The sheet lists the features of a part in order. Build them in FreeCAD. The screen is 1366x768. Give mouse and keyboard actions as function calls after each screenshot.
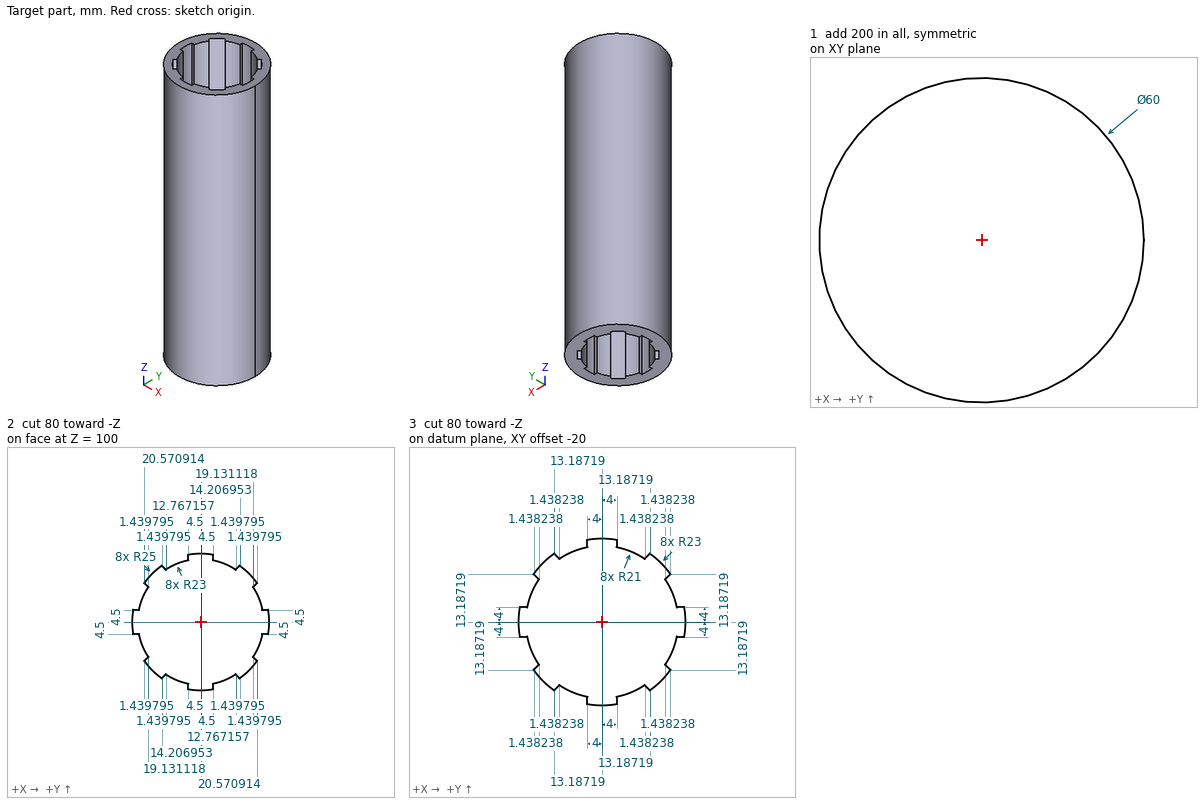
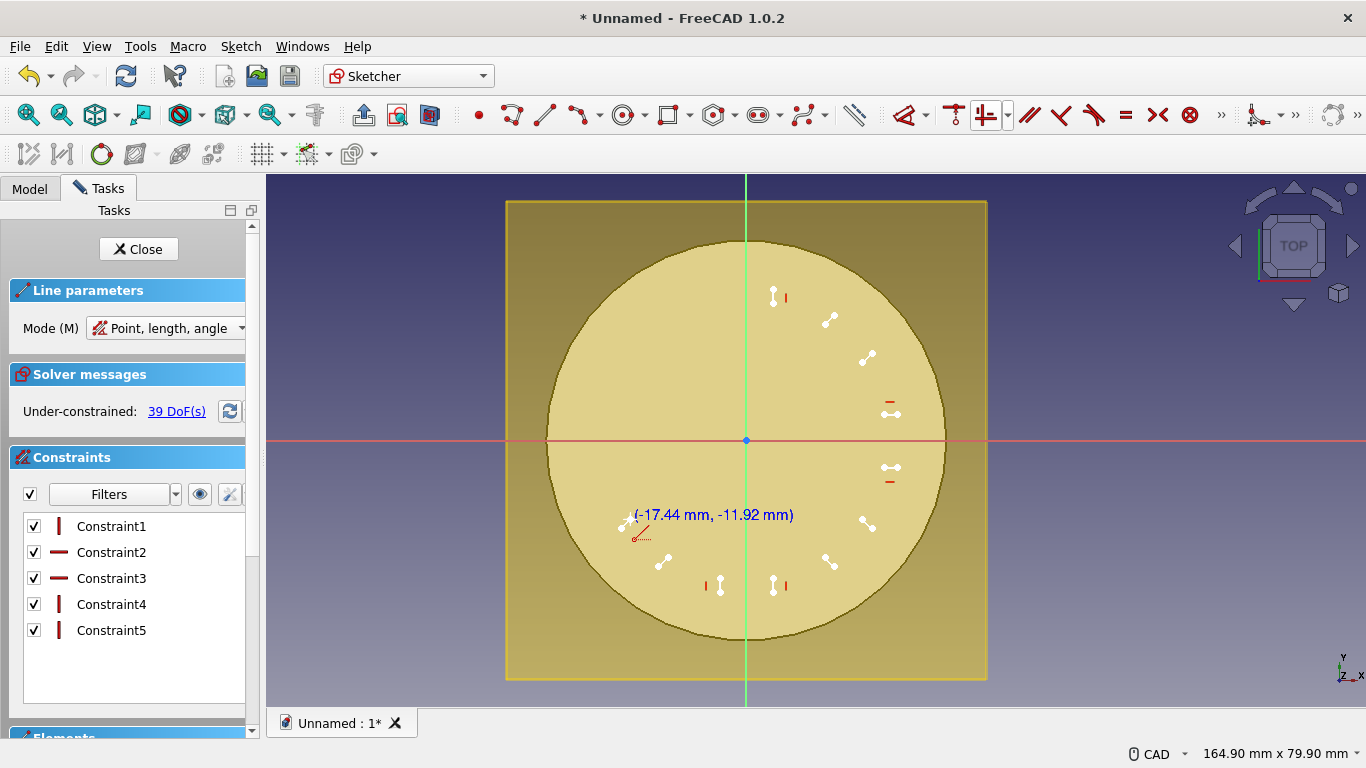
click(609, 467)
click(595, 467)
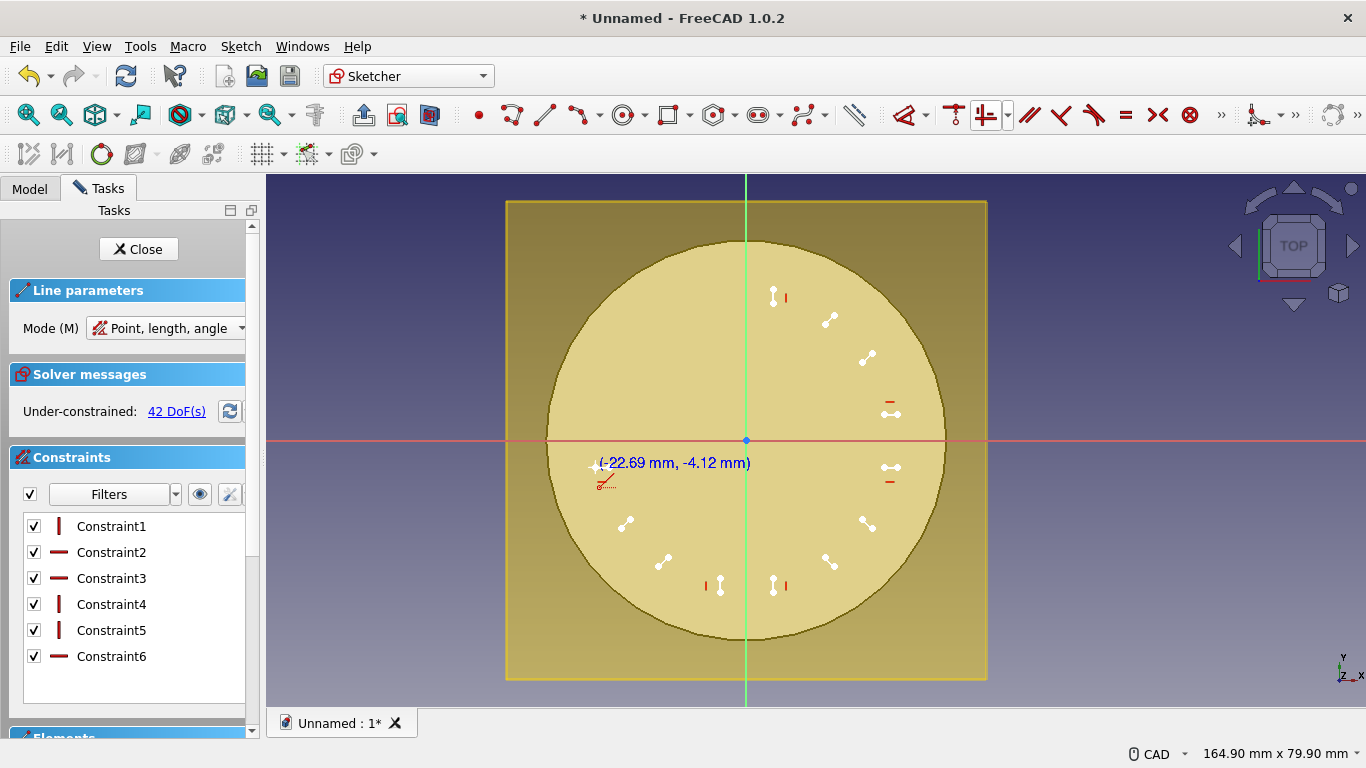
click(595, 414)
click(609, 414)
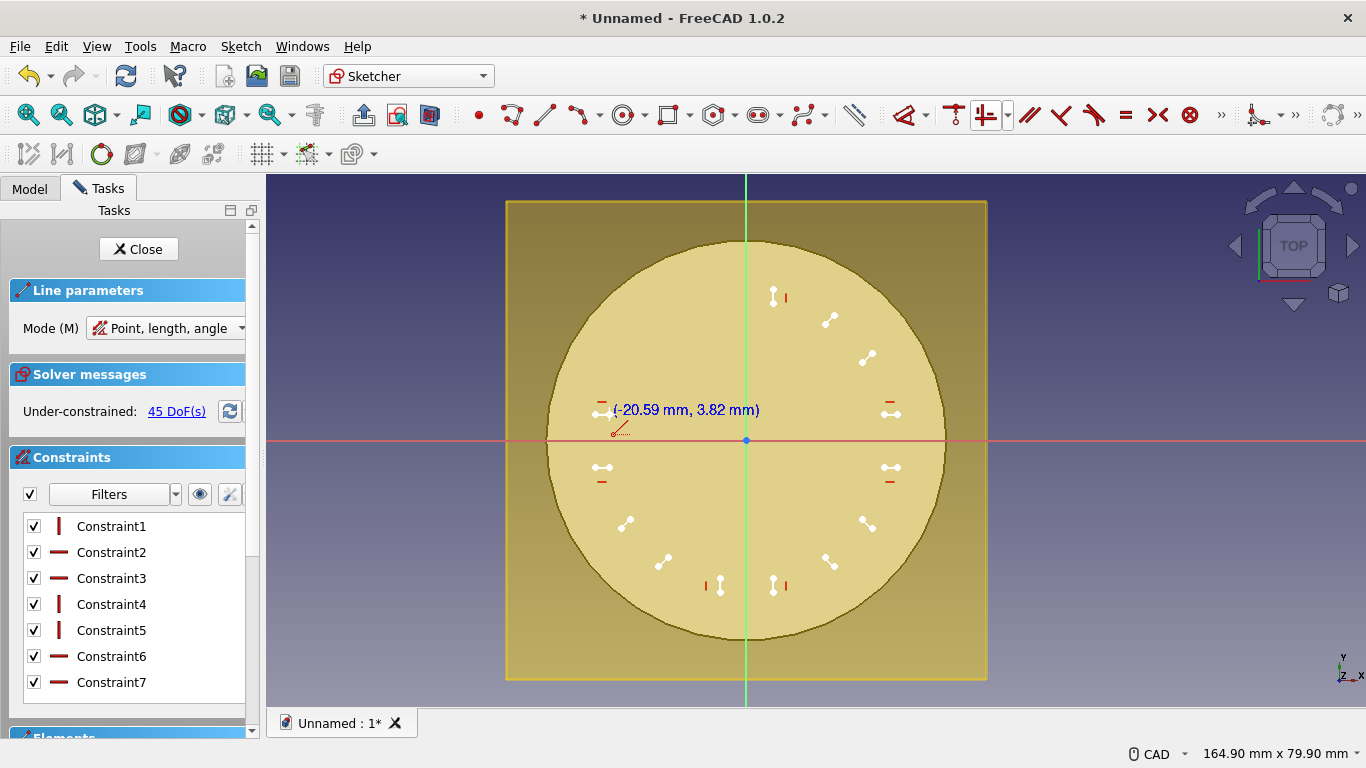
click(630, 362)
click(621, 353)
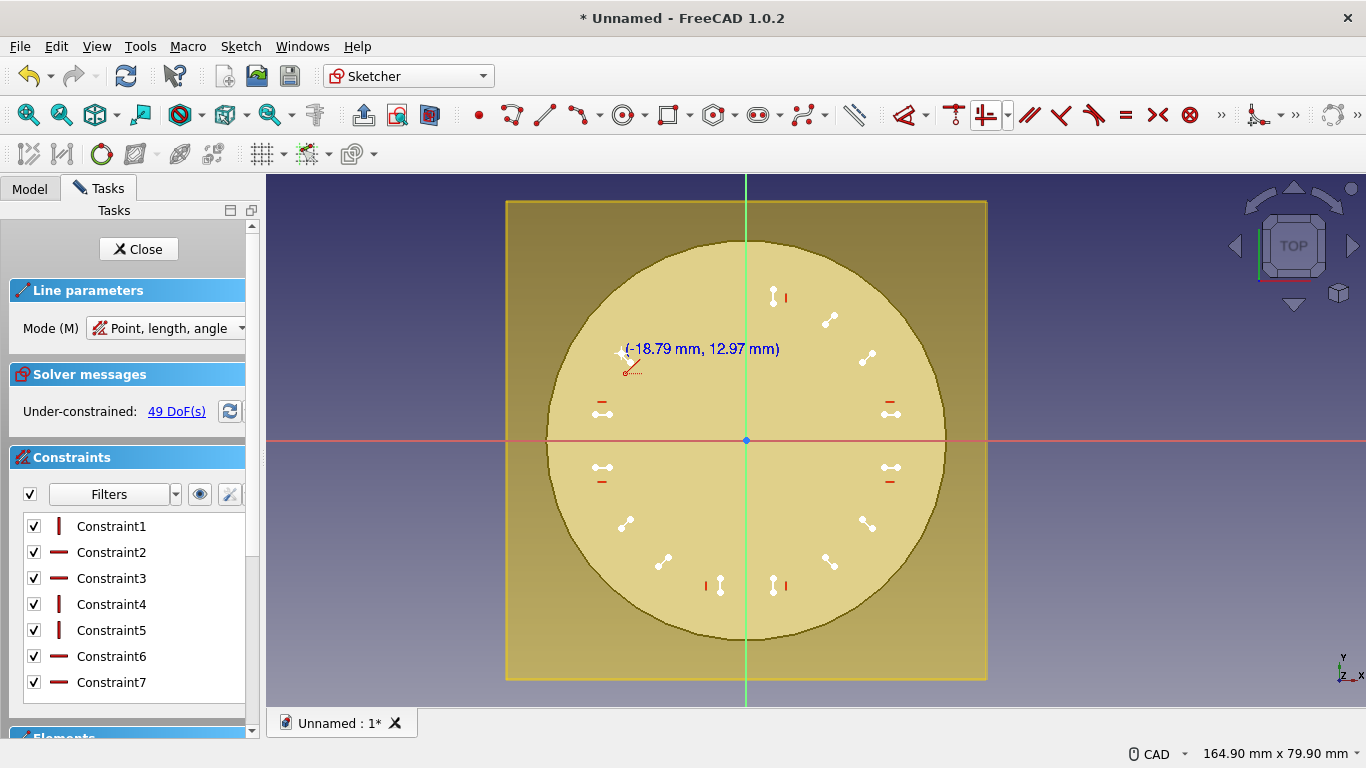
click(658, 315)
click(668, 324)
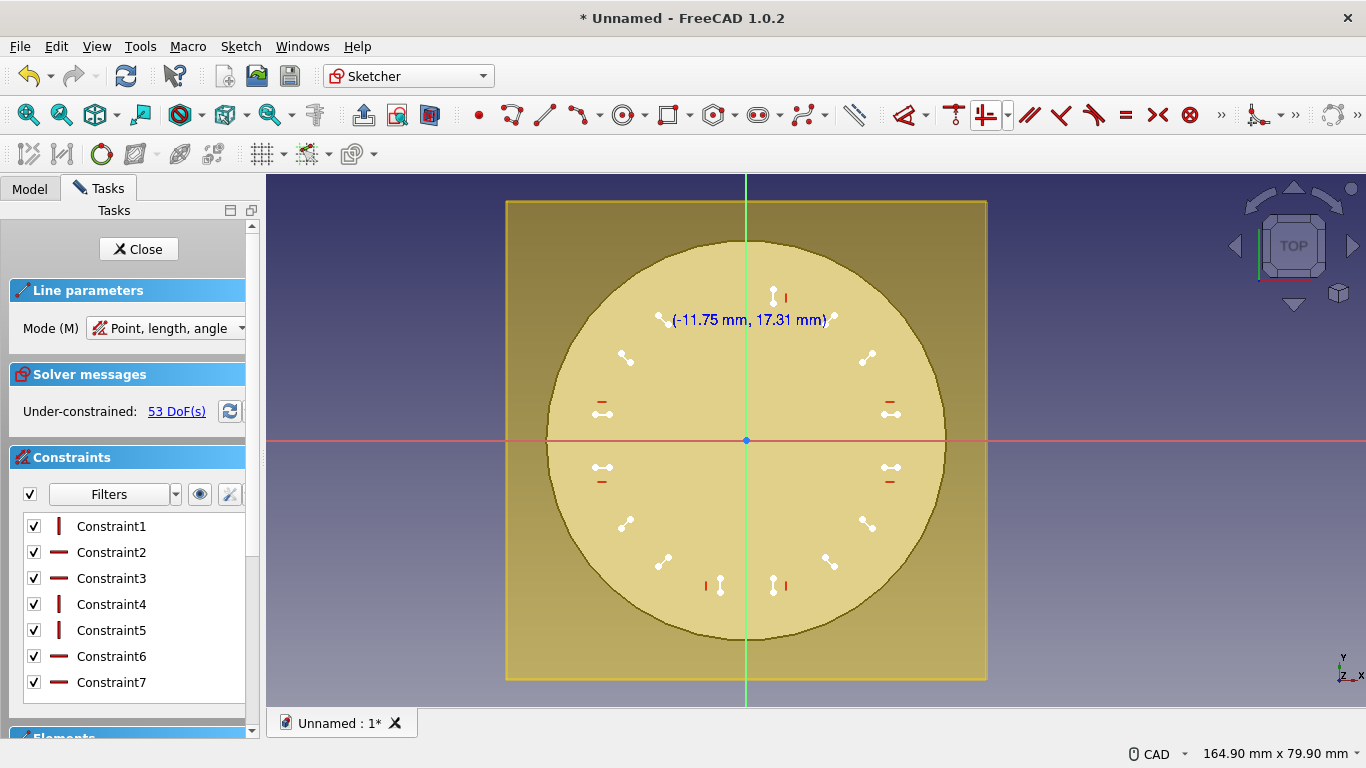
click(720, 303)
click(720, 289)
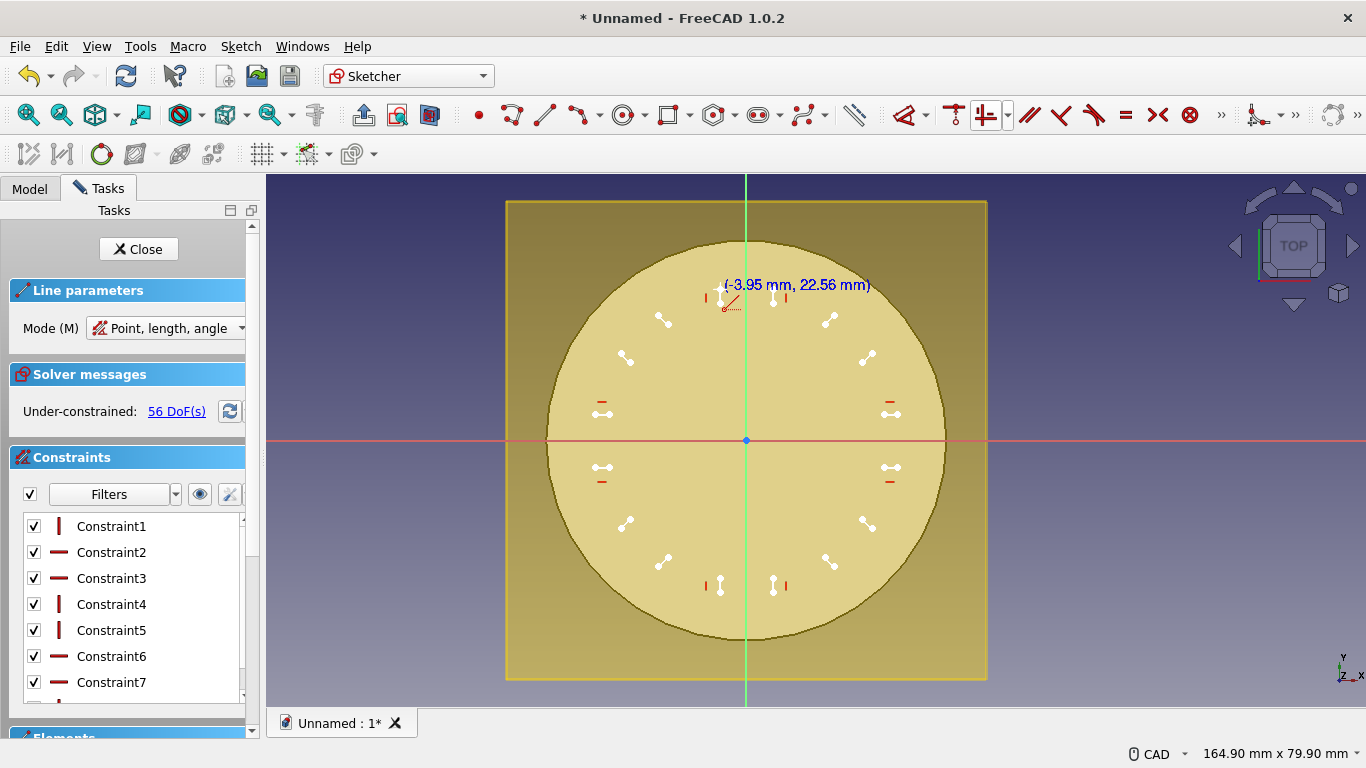
click(578, 116)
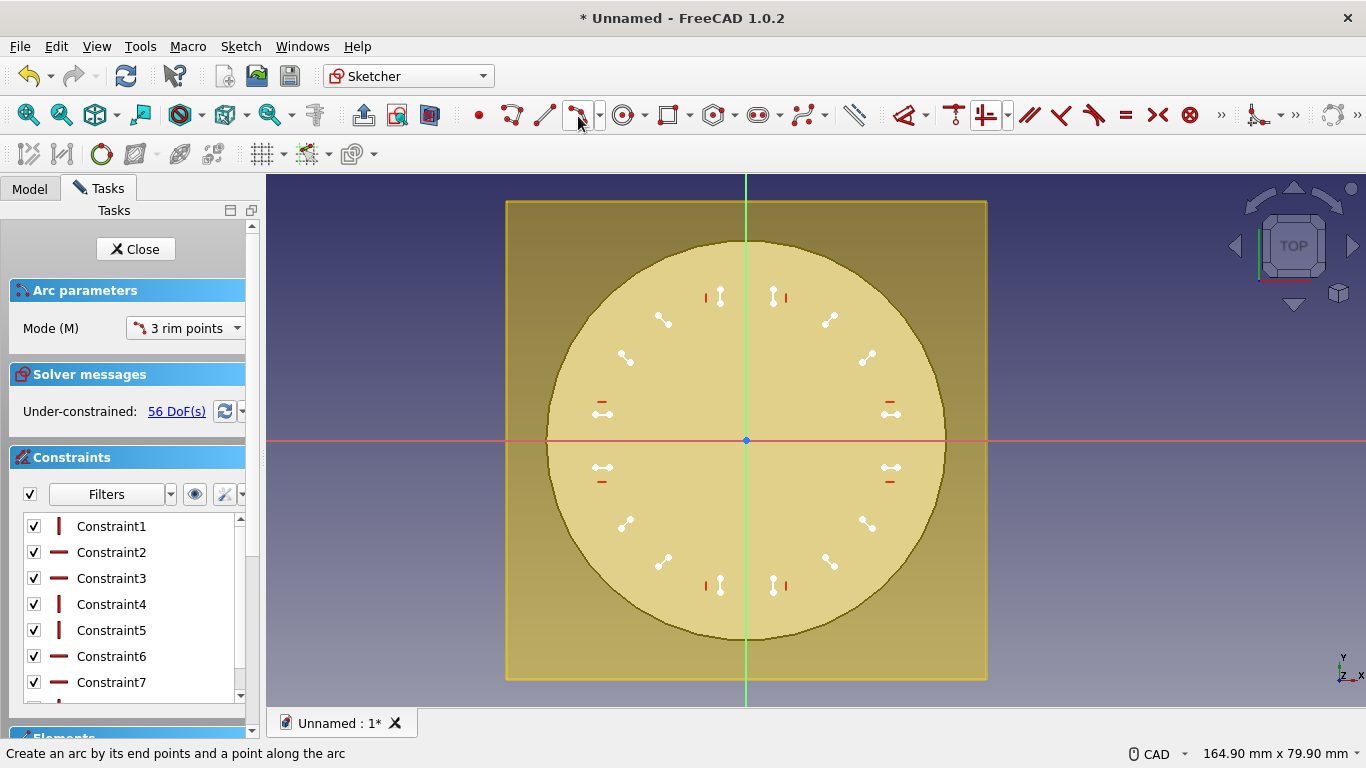
scroll(773, 303, up, 5)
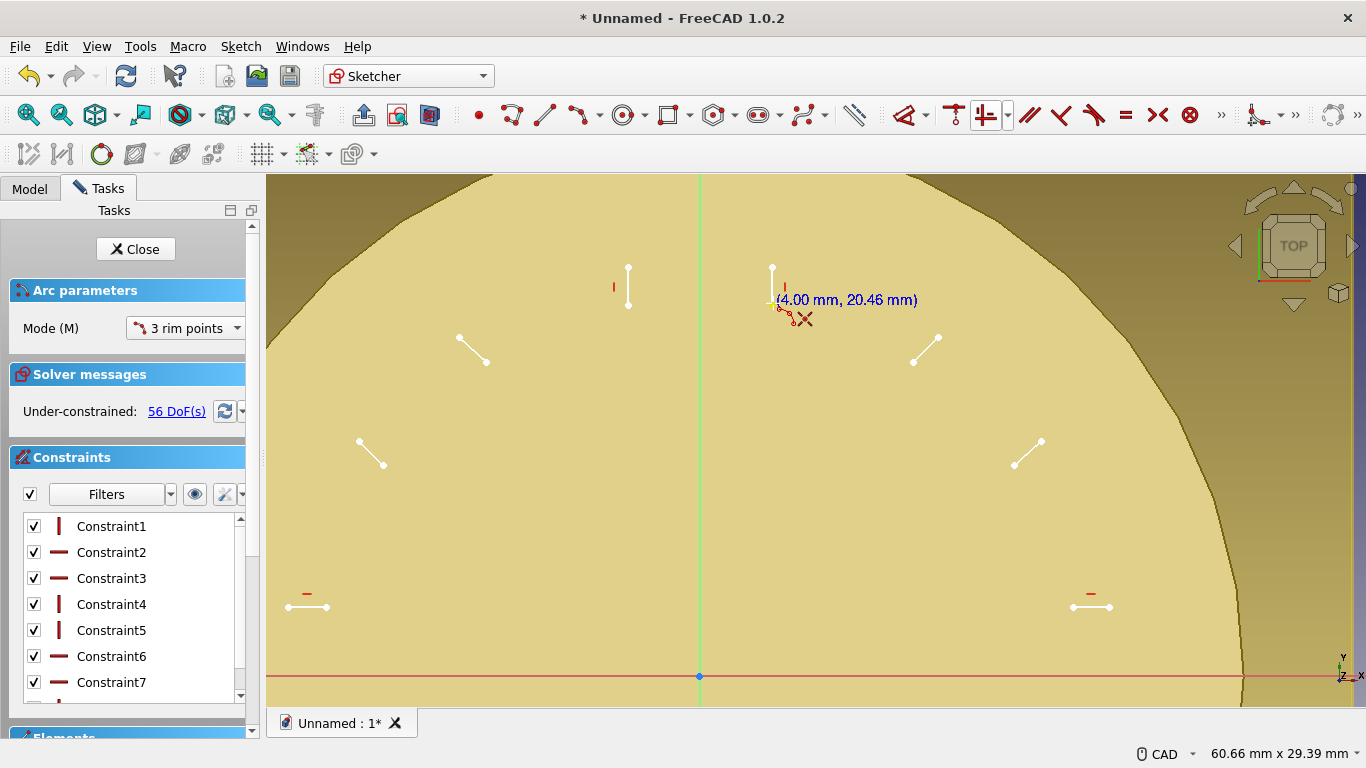
click(772, 305)
click(914, 362)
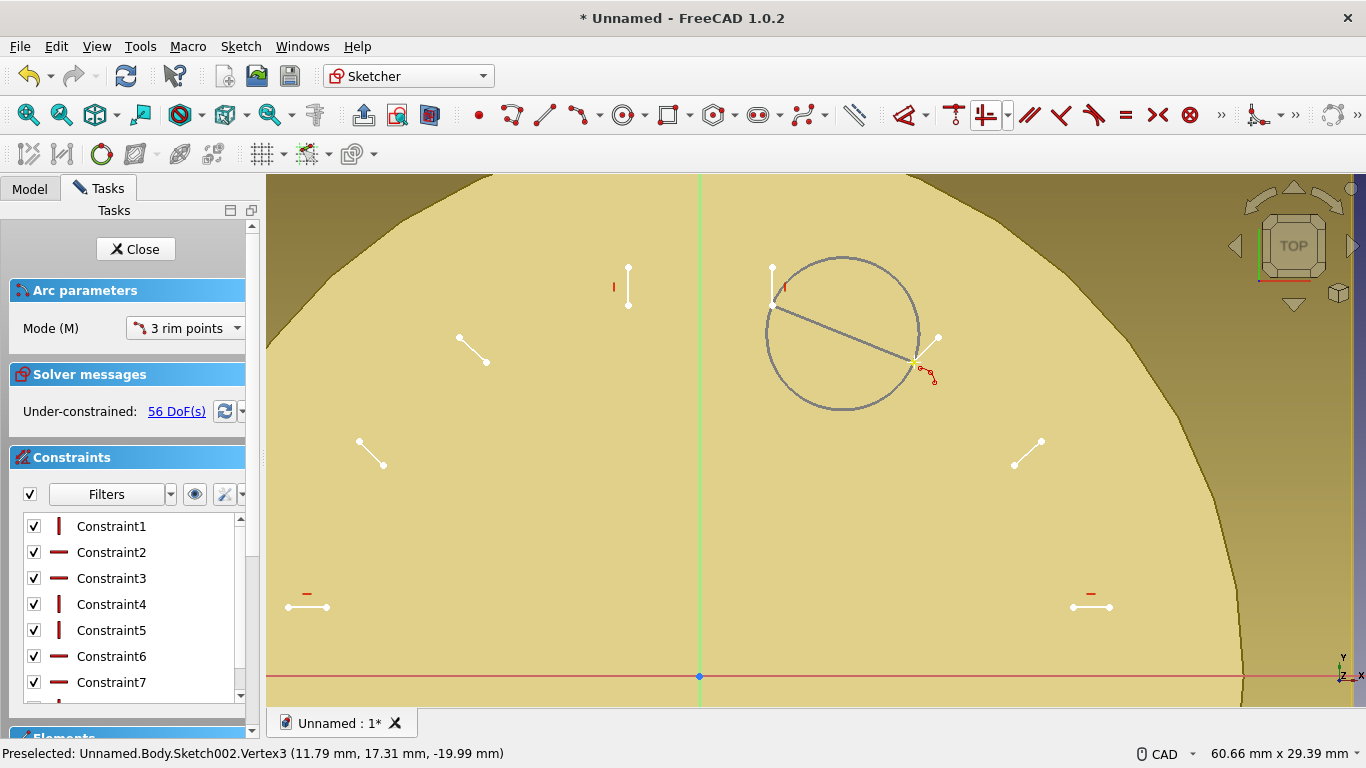
scroll(845, 325, up, 4)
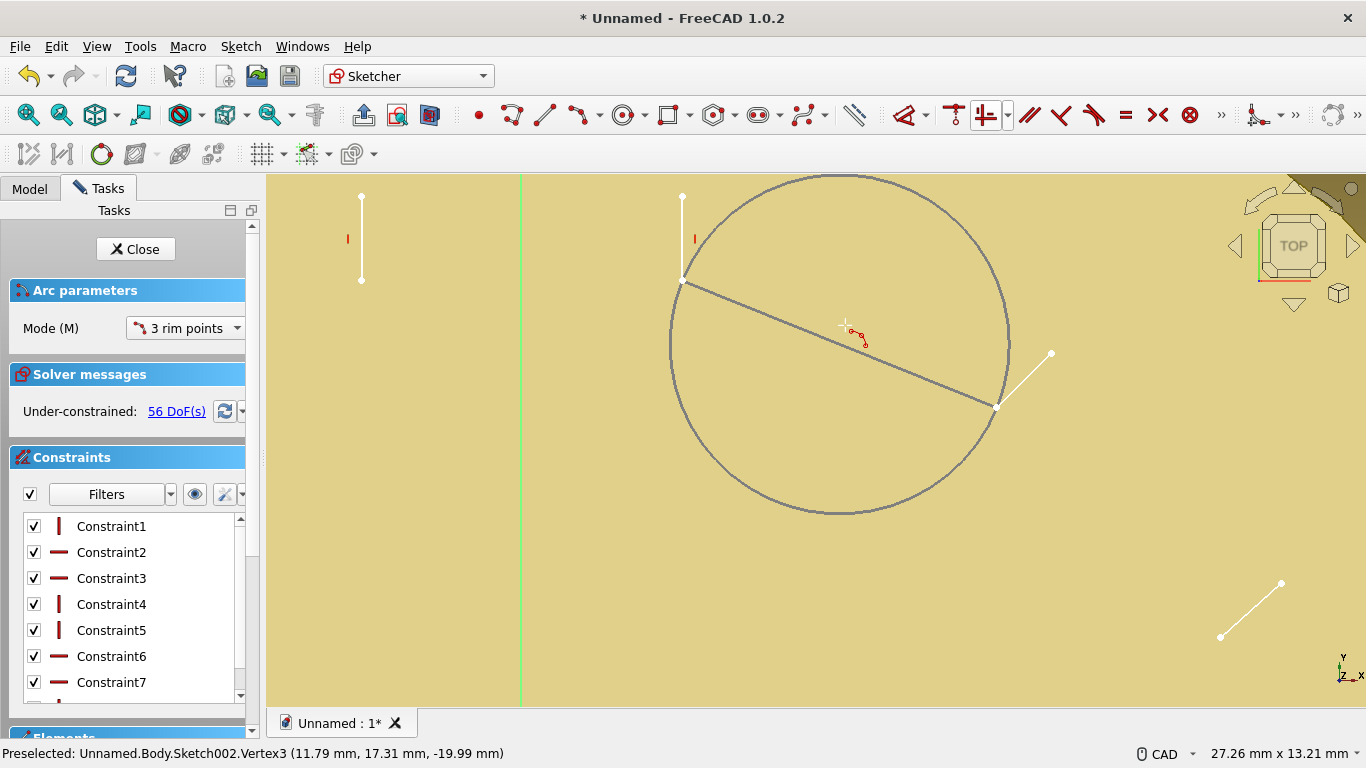
click(845, 324)